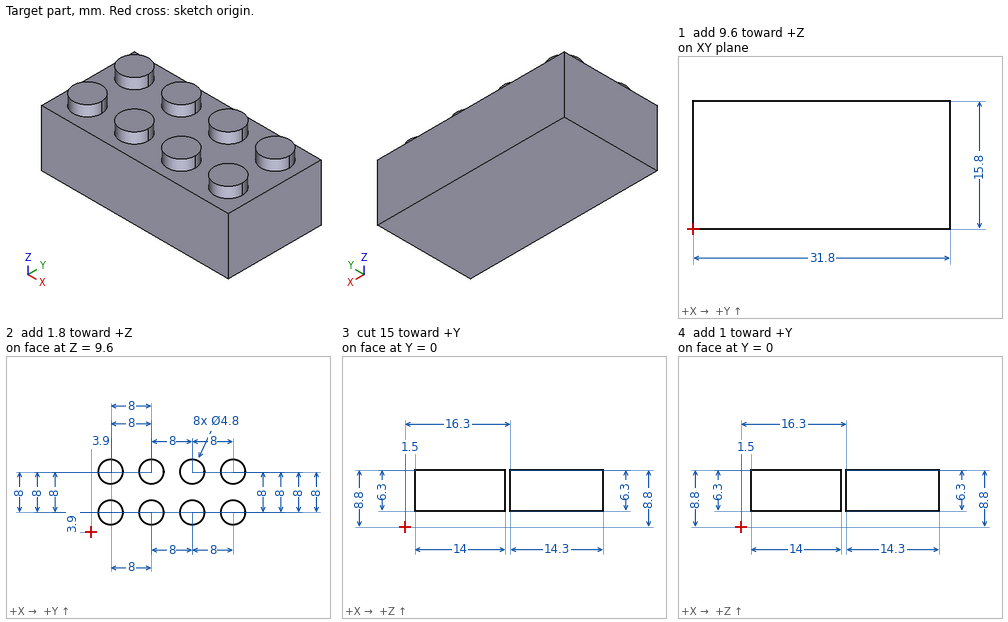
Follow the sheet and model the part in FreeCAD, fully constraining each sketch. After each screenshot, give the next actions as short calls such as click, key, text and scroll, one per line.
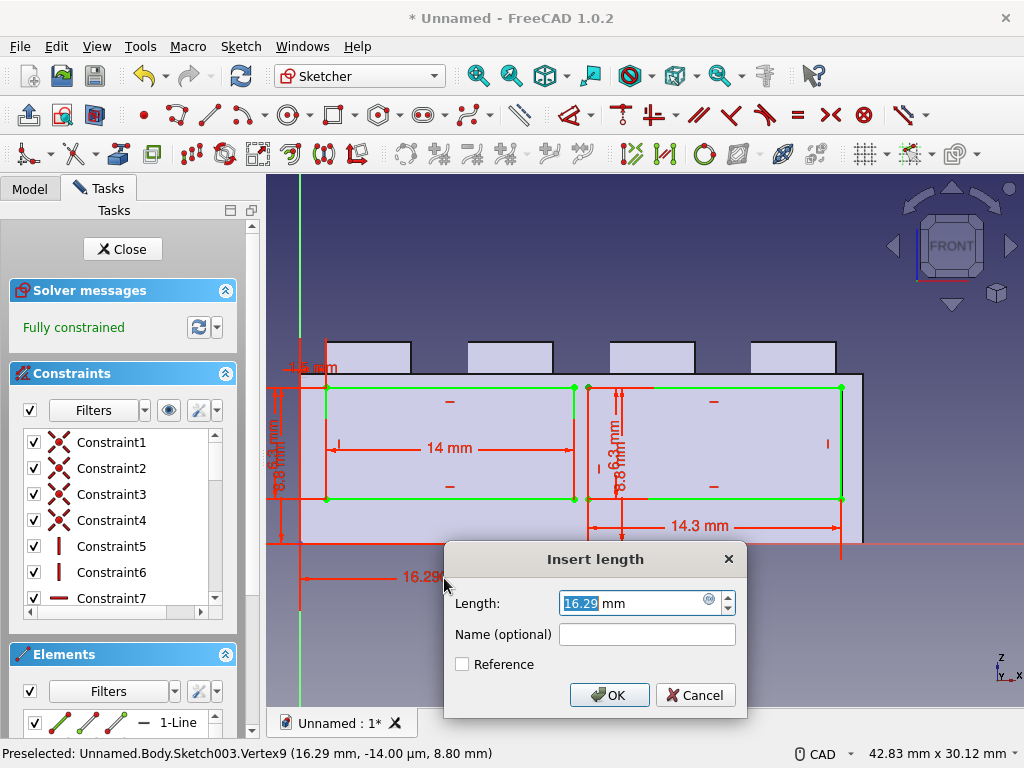
text(16.3)
key(Return)
key(Escape)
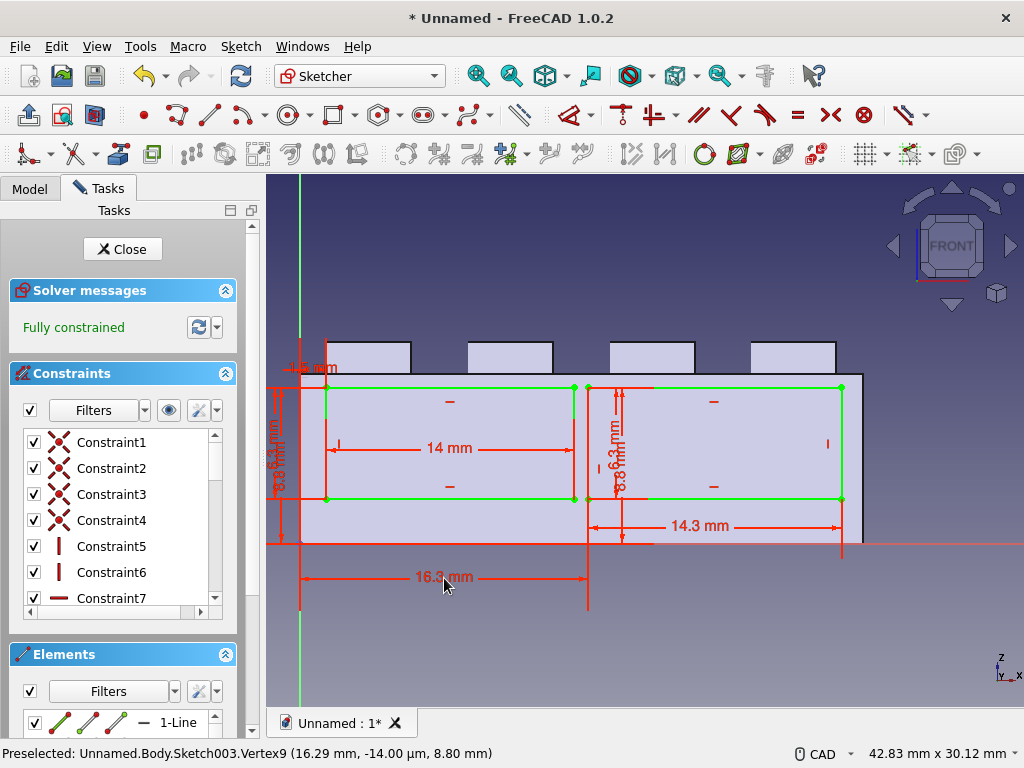
click(123, 249)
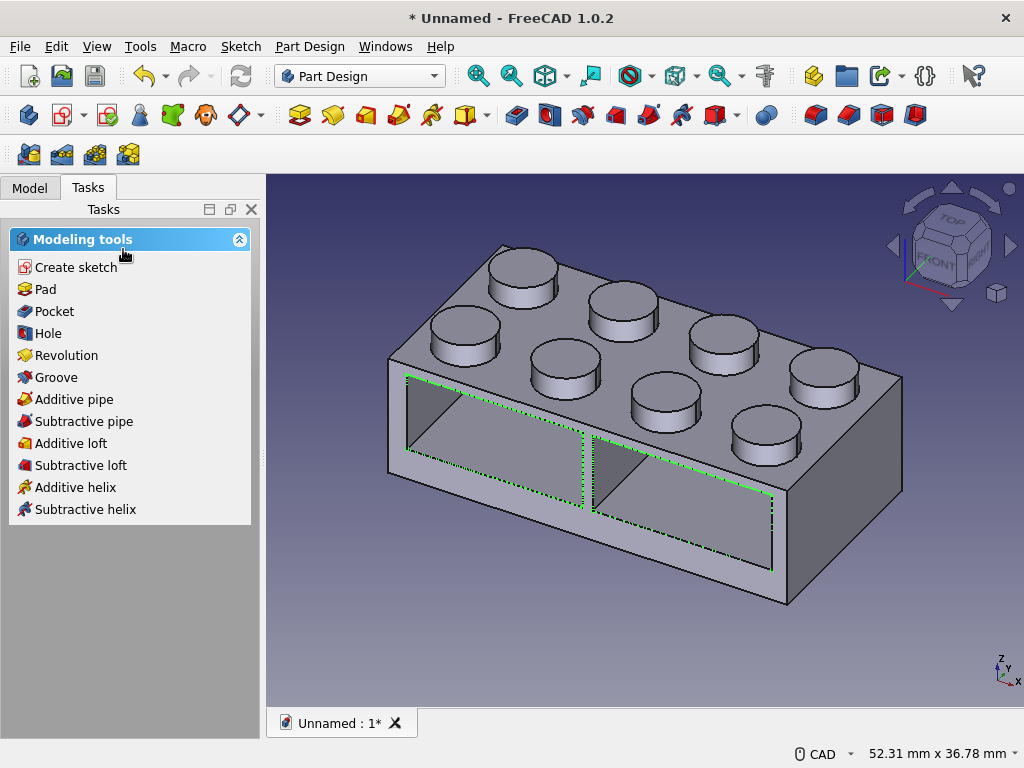
click(300, 116)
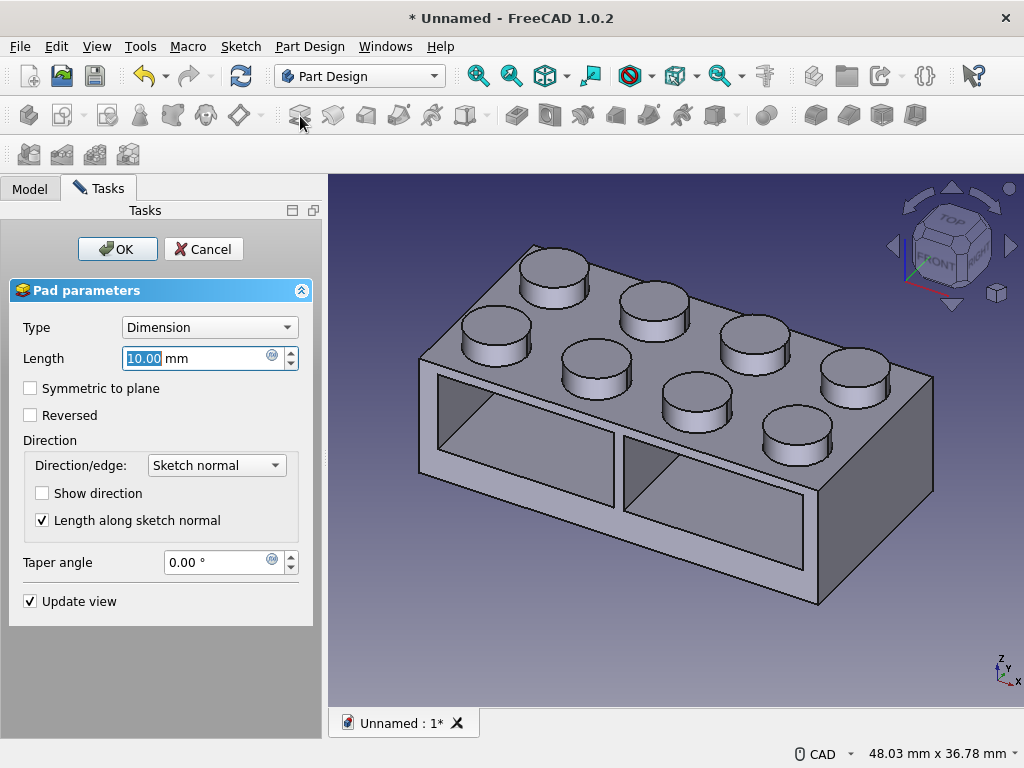
text(1)
key(Tab)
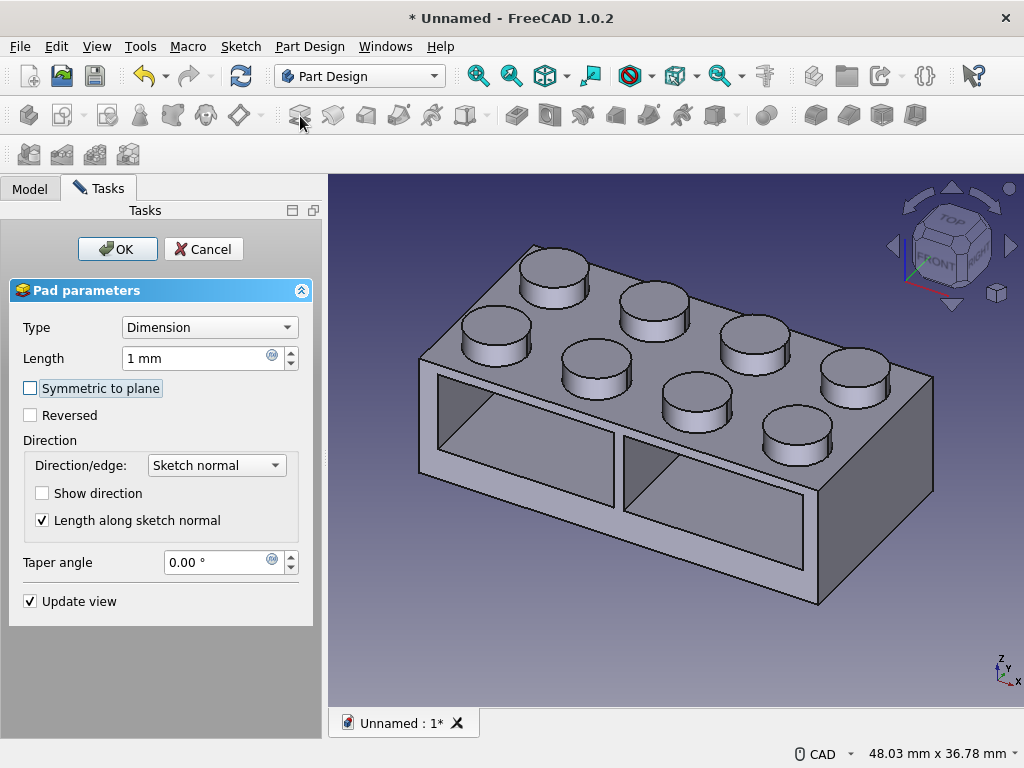
click(31, 415)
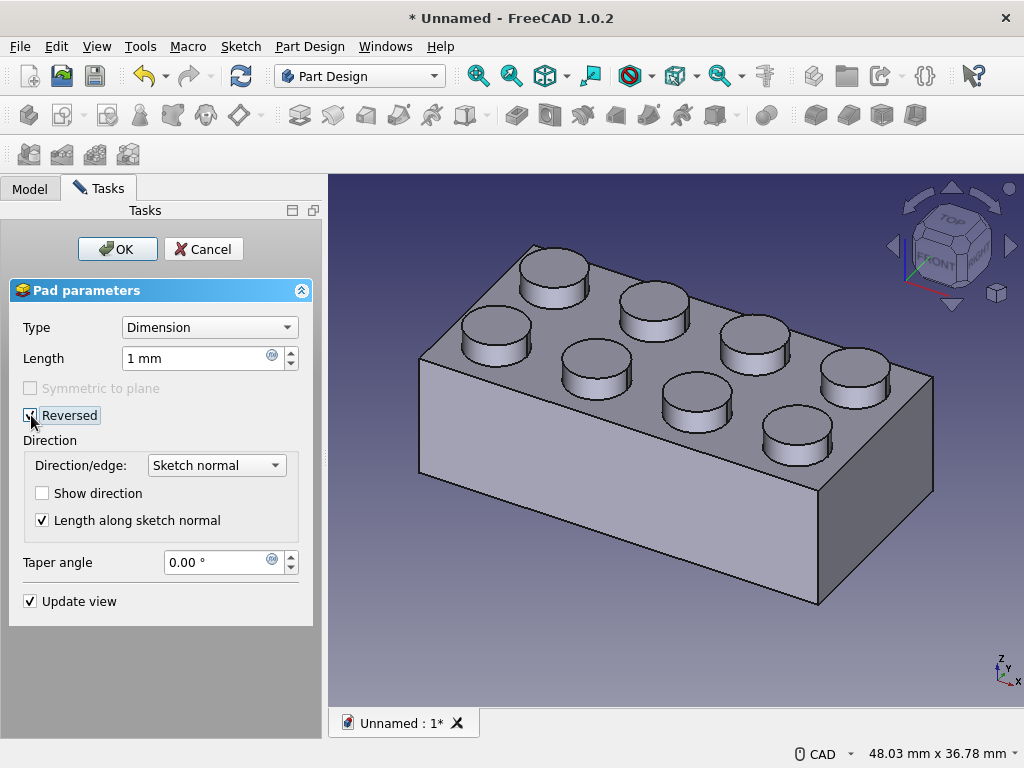
click(118, 249)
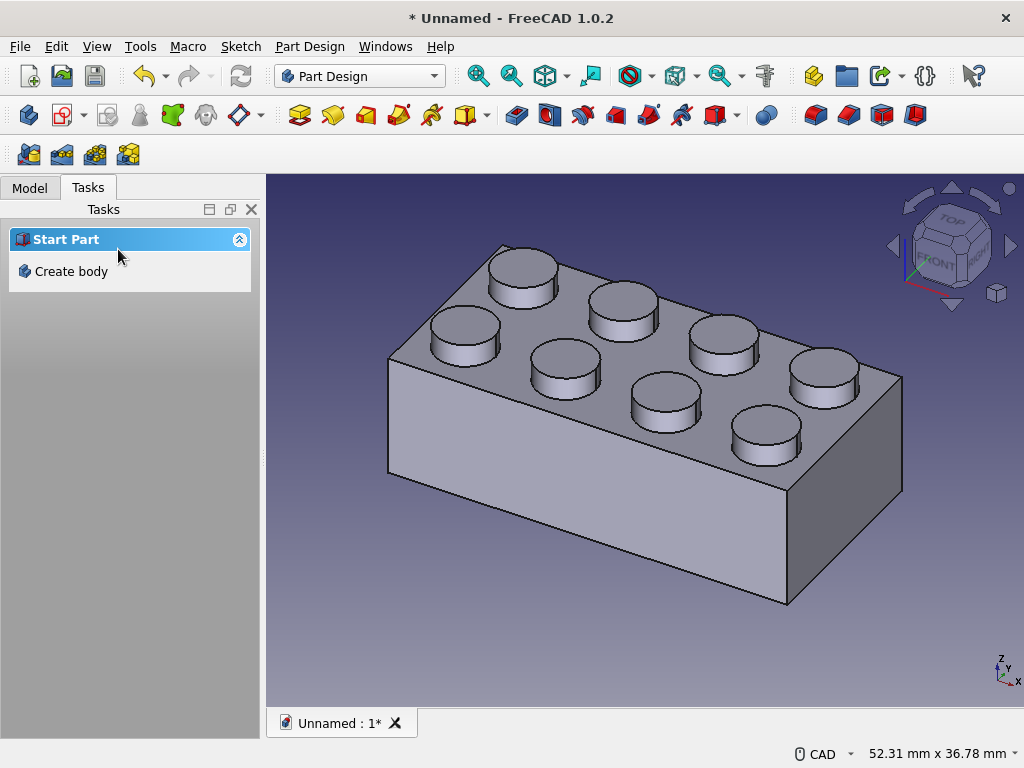
key(0)